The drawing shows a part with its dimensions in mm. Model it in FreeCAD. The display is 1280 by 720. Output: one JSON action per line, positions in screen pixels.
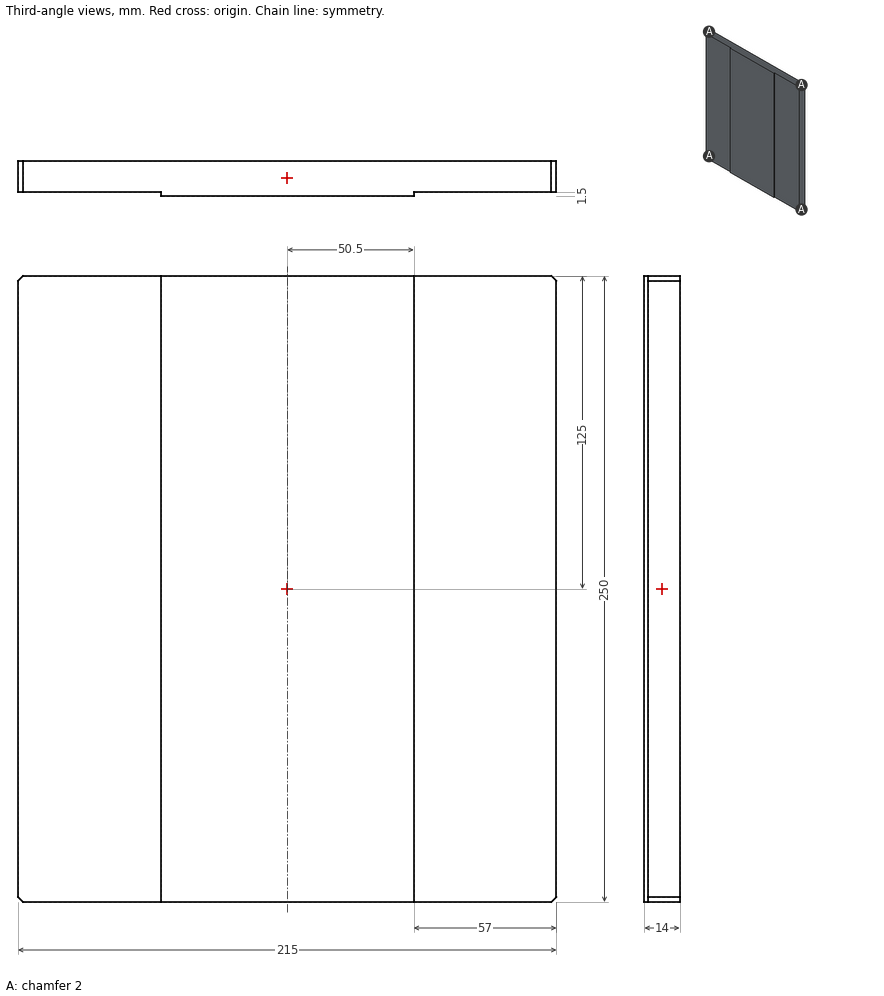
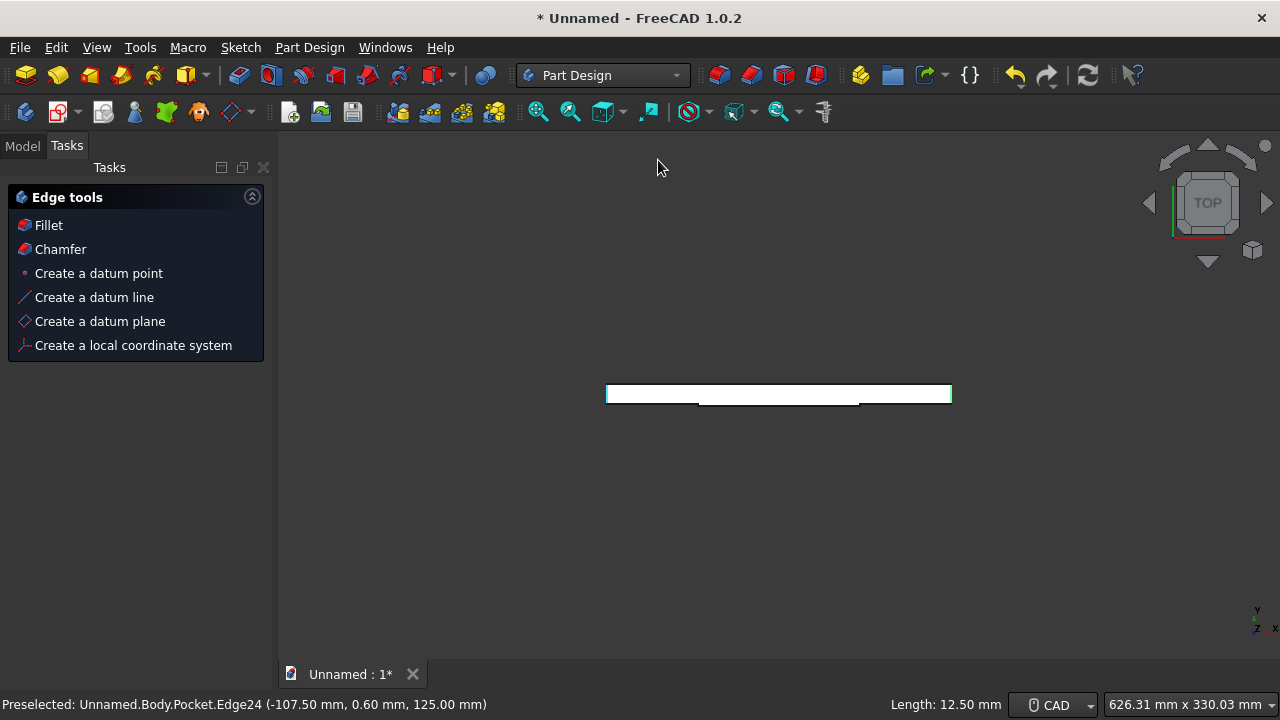
{"action": "key", "text": "v f"}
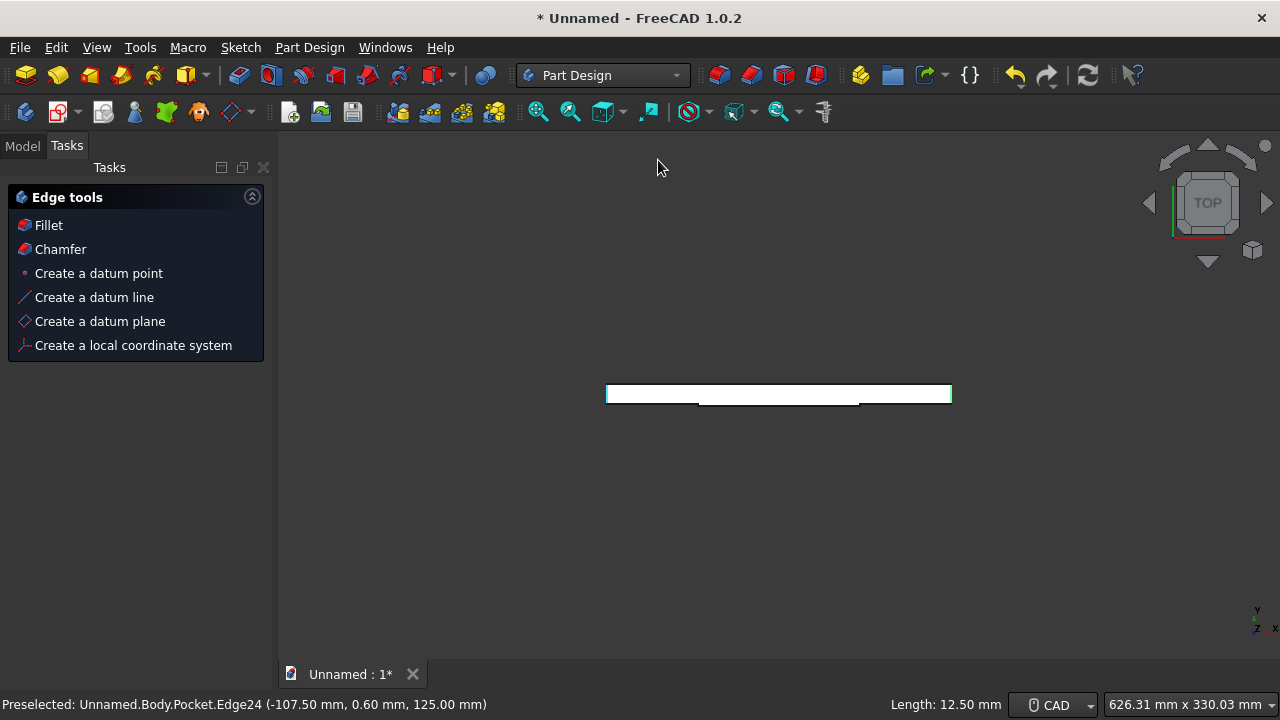
{"action": "left_click", "coordinate": [607, 393], "text": "ctrl"}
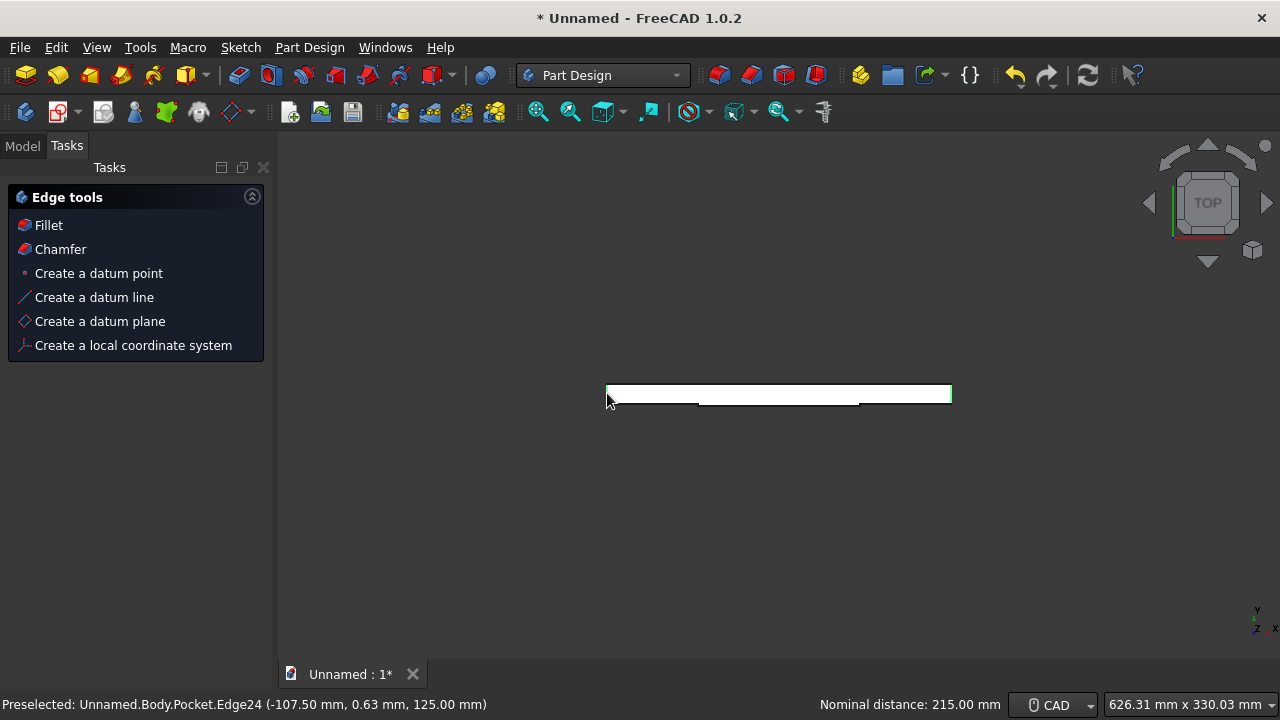
{"action": "scroll", "coordinate": [607, 393], "scroll_direction": "up", "scroll_amount": 4}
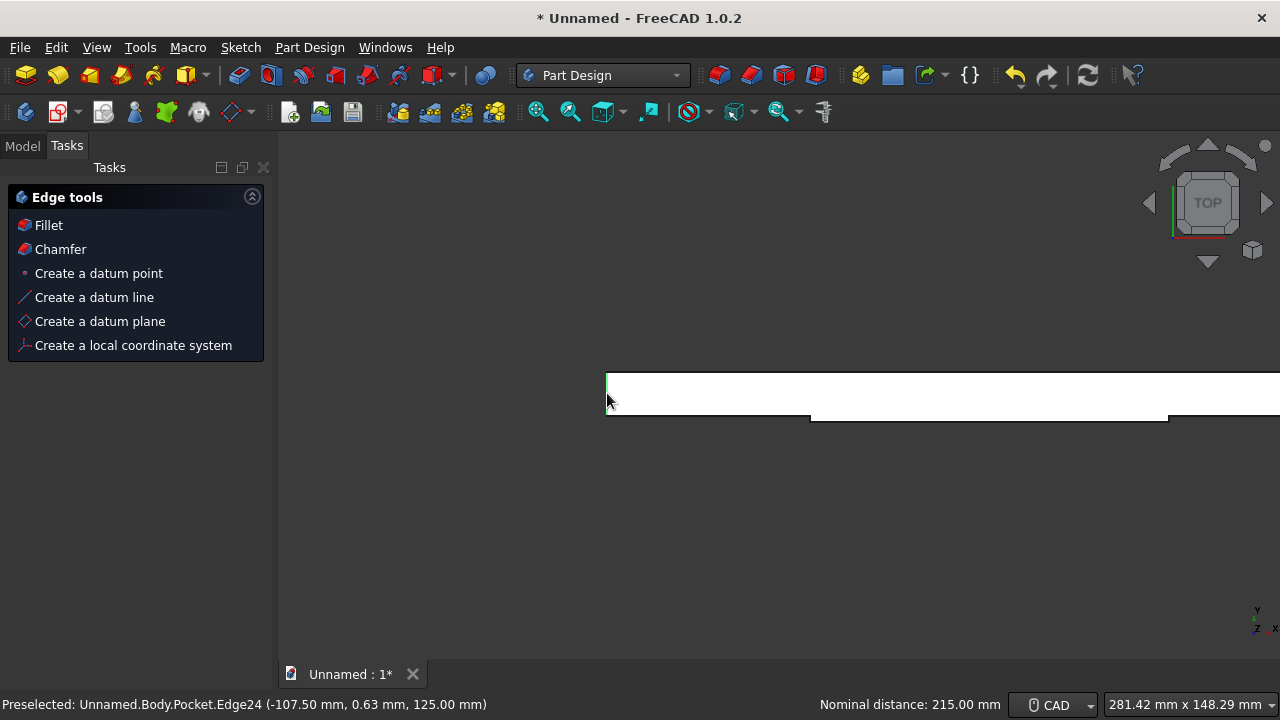
{"action": "left_click", "coordinate": [540, 112]}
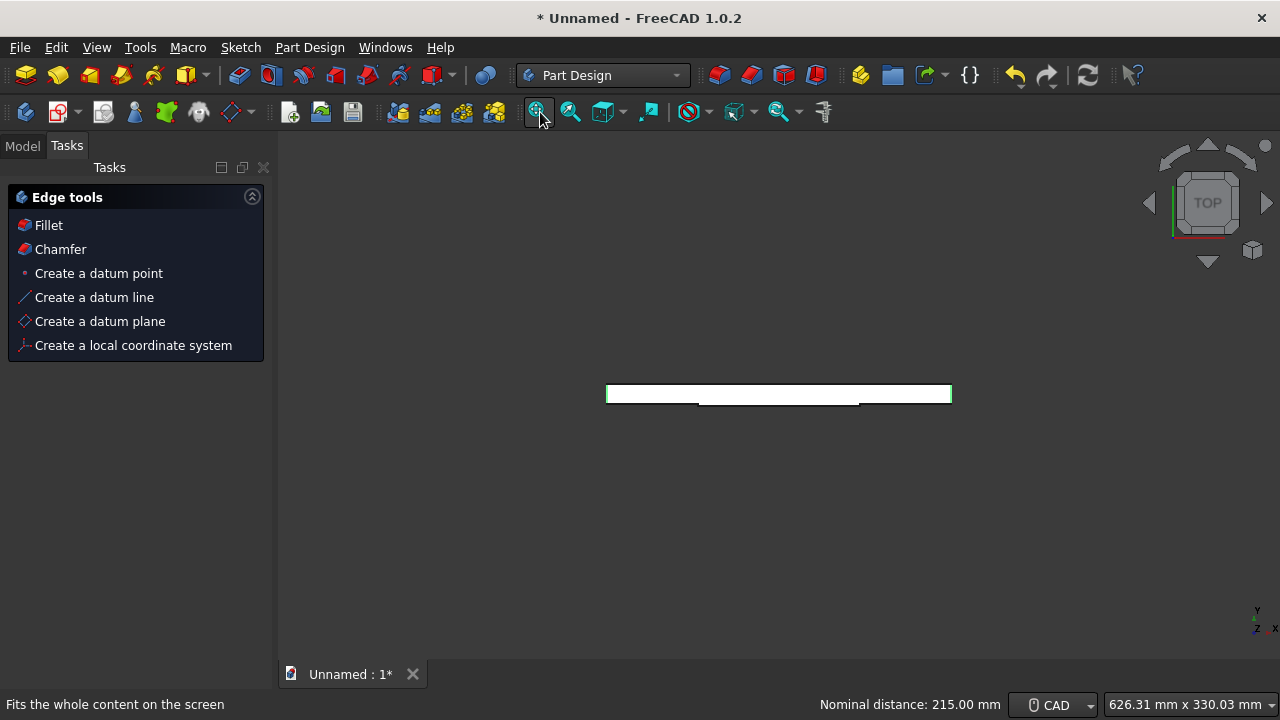
{"action": "key", "text": "1"}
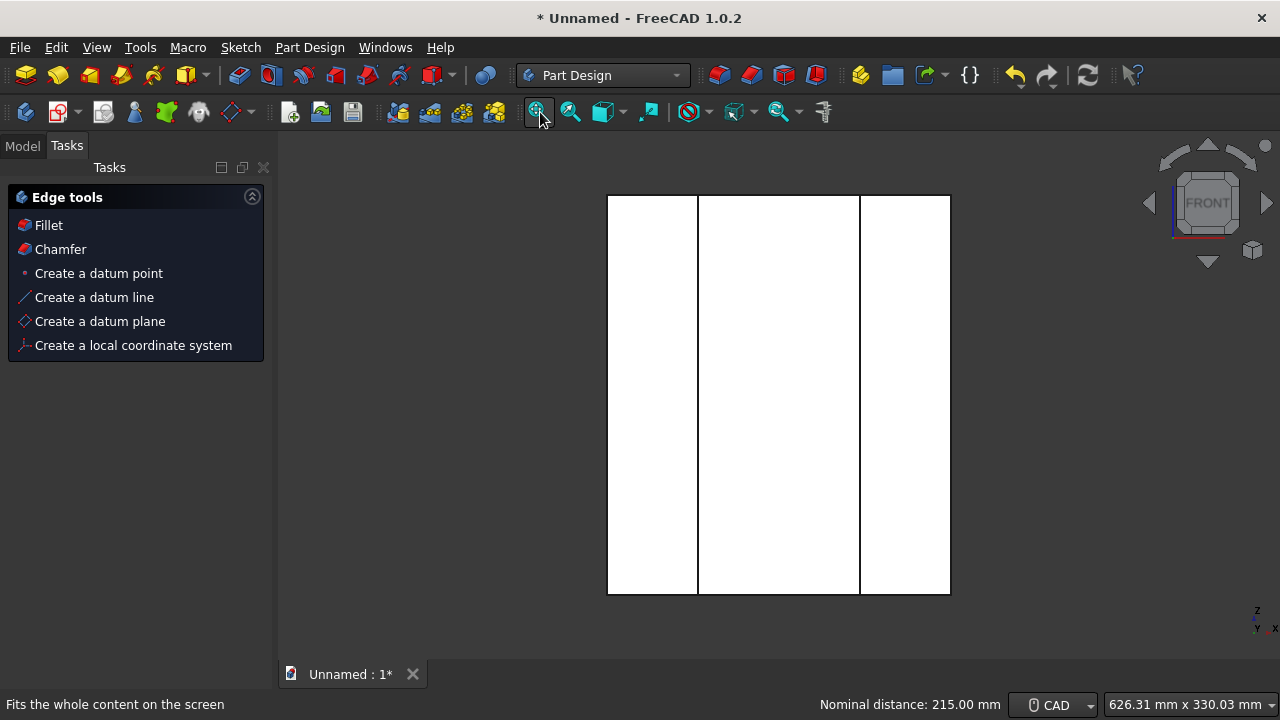
{"action": "scroll", "coordinate": [607, 594], "scroll_direction": "up", "scroll_amount": 4}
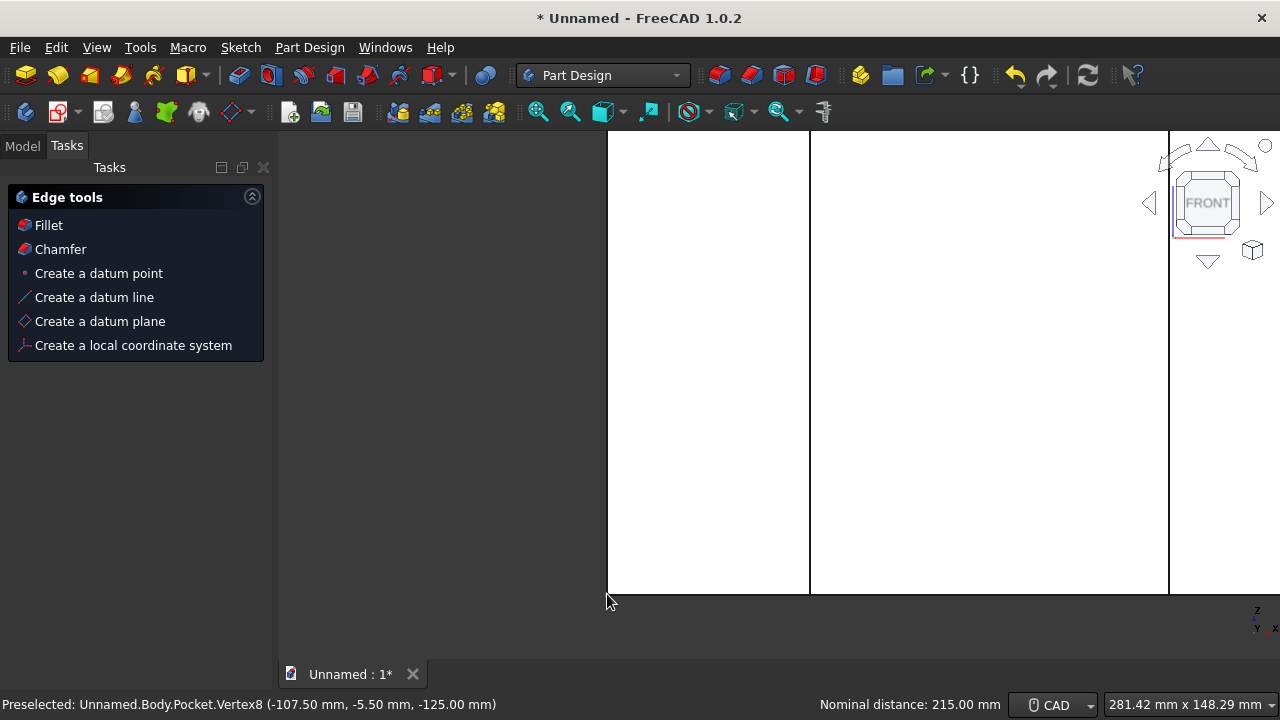
{"action": "key", "text": "v f"}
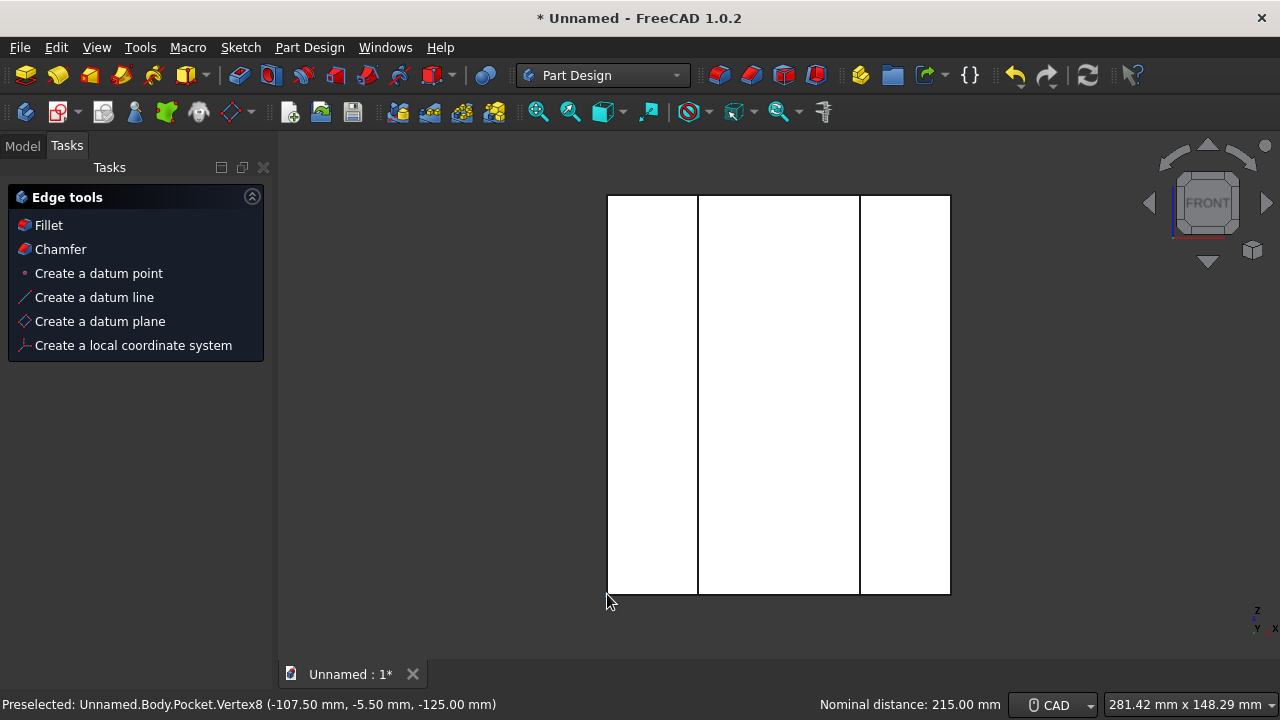
{"action": "key", "text": "3"}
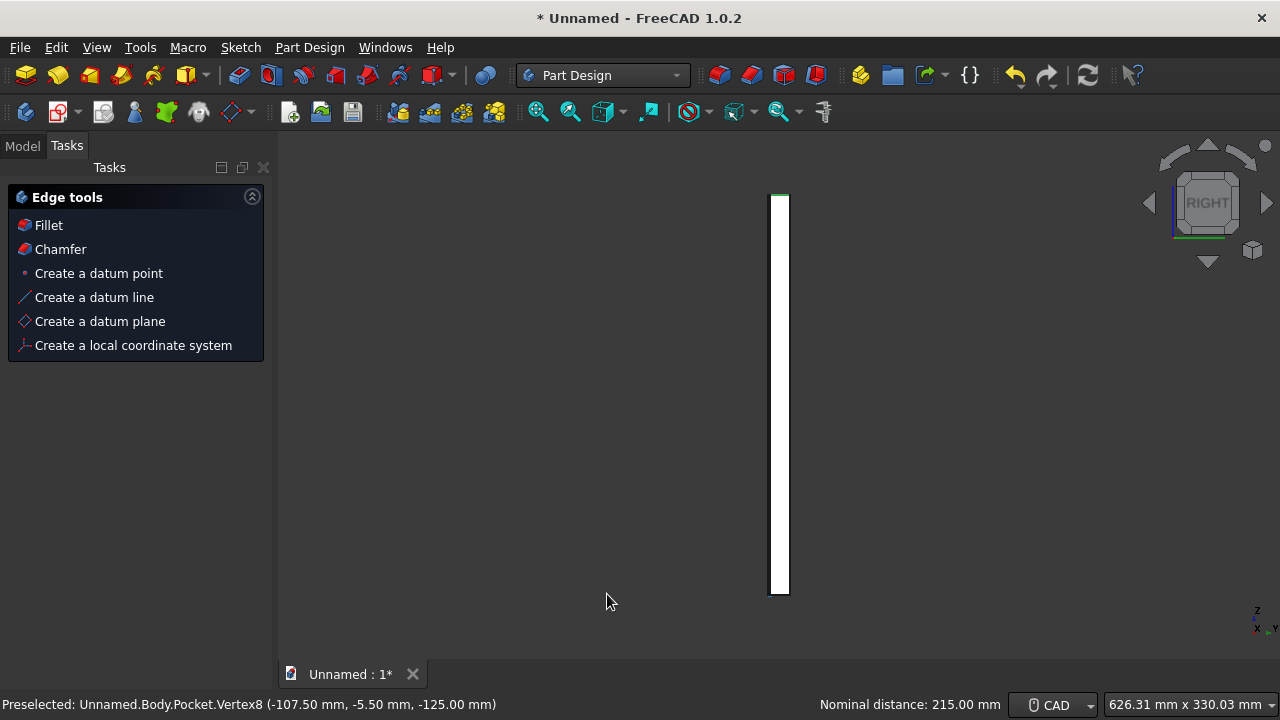
{"action": "left_click", "coordinate": [780, 594], "text": "ctrl"}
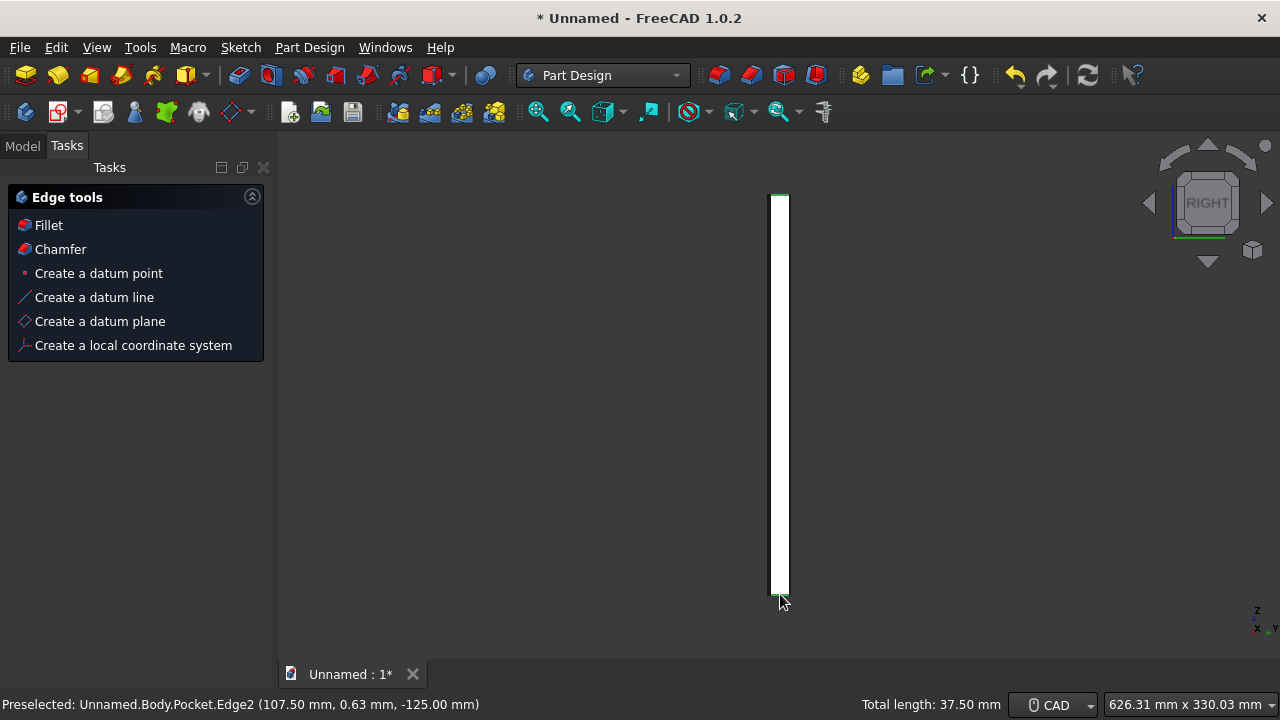
{"action": "scroll", "coordinate": [780, 594], "scroll_direction": "up", "scroll_amount": 4}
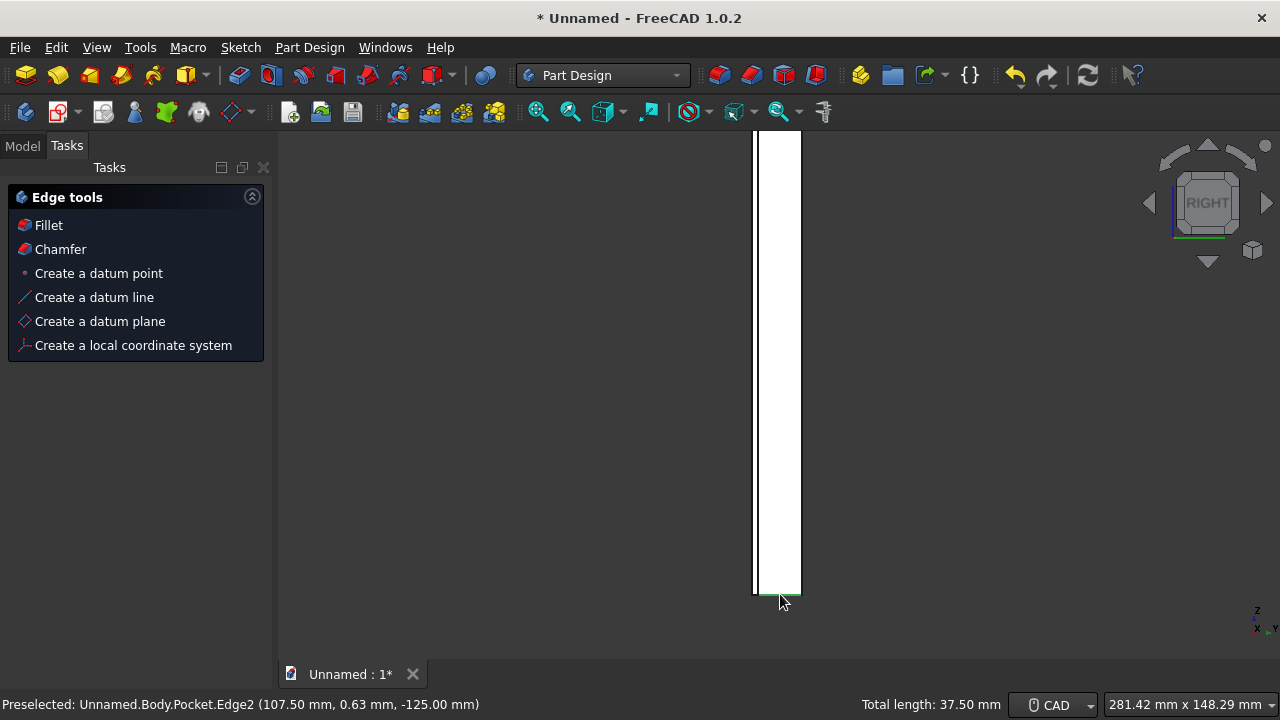
{"action": "key", "text": "v f"}